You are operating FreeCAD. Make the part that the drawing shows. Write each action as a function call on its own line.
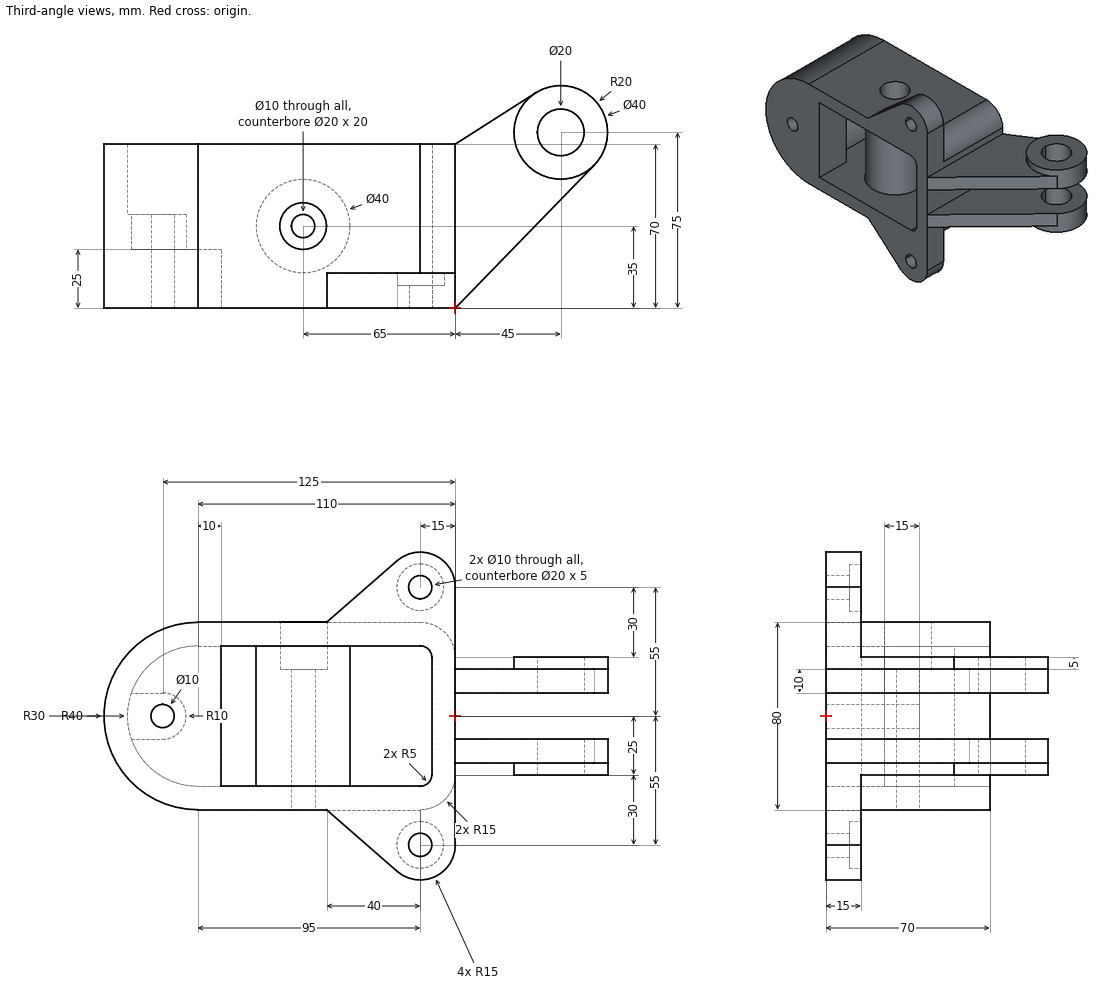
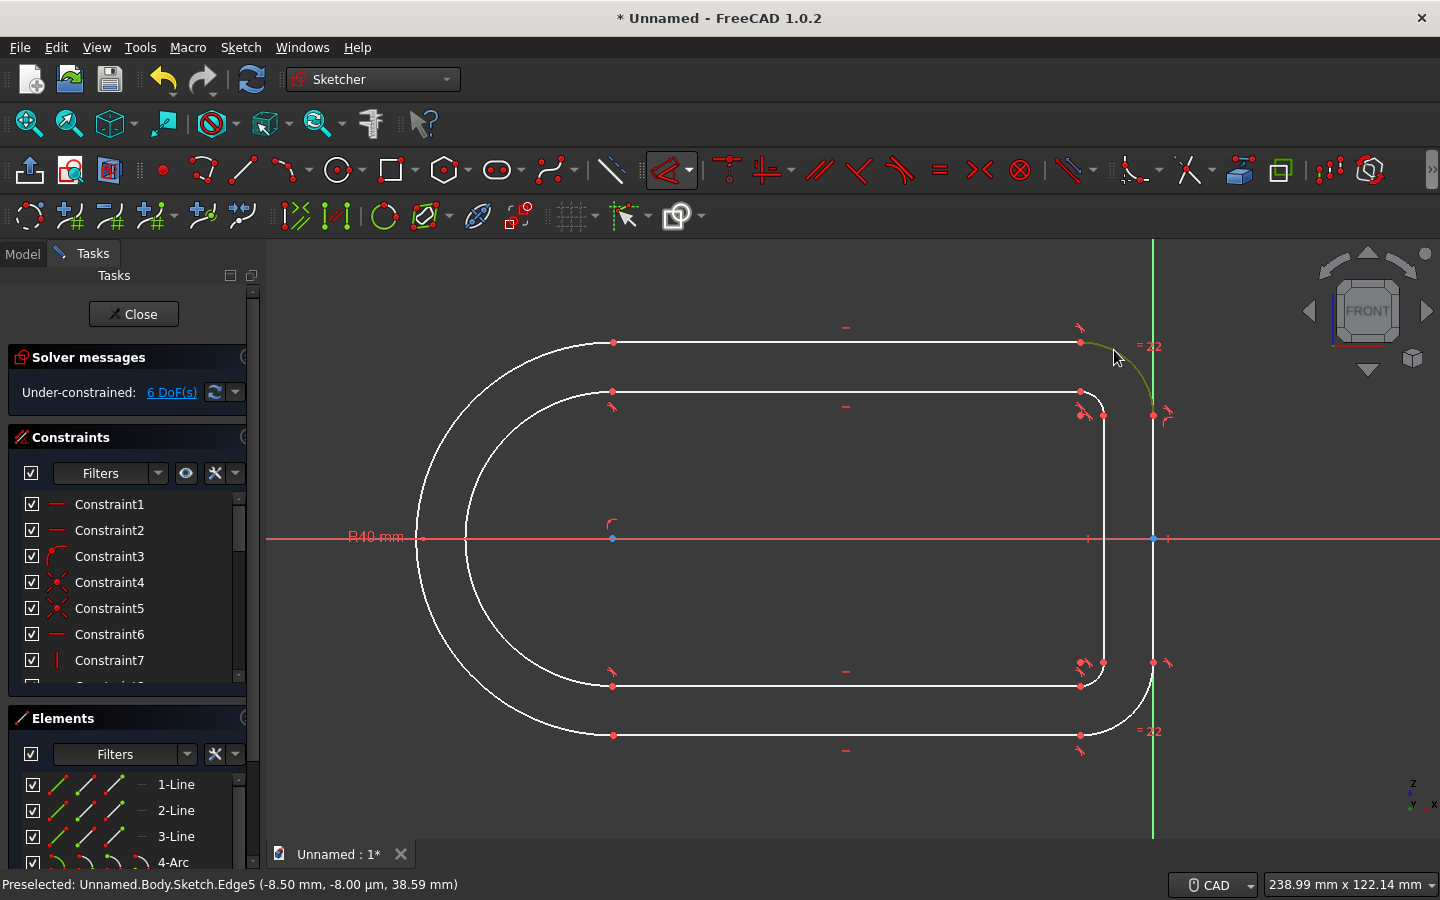
key(k)
key(r)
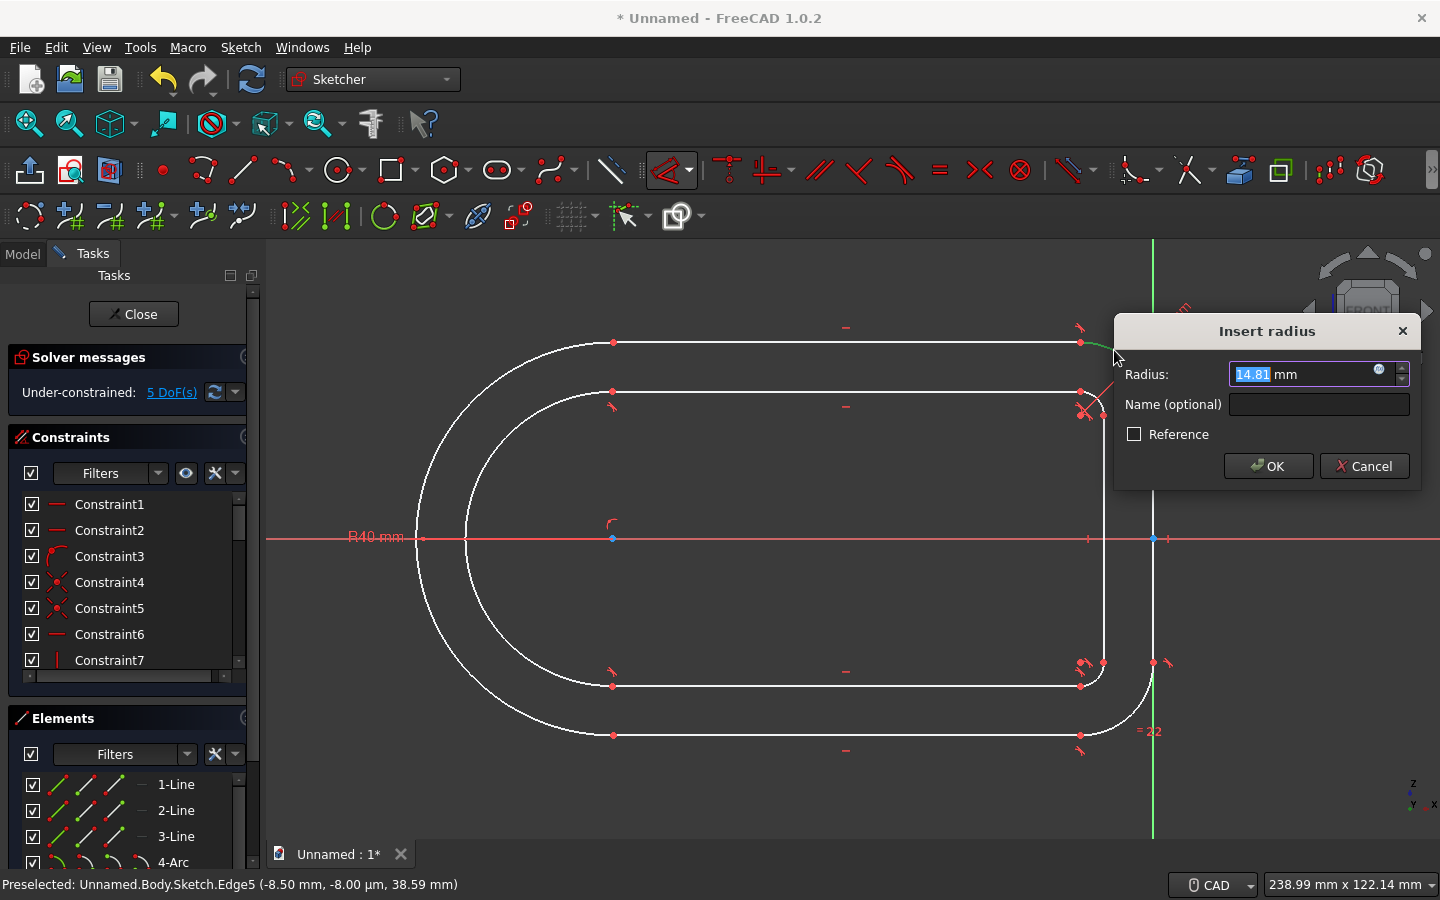
text(15)
key(Return)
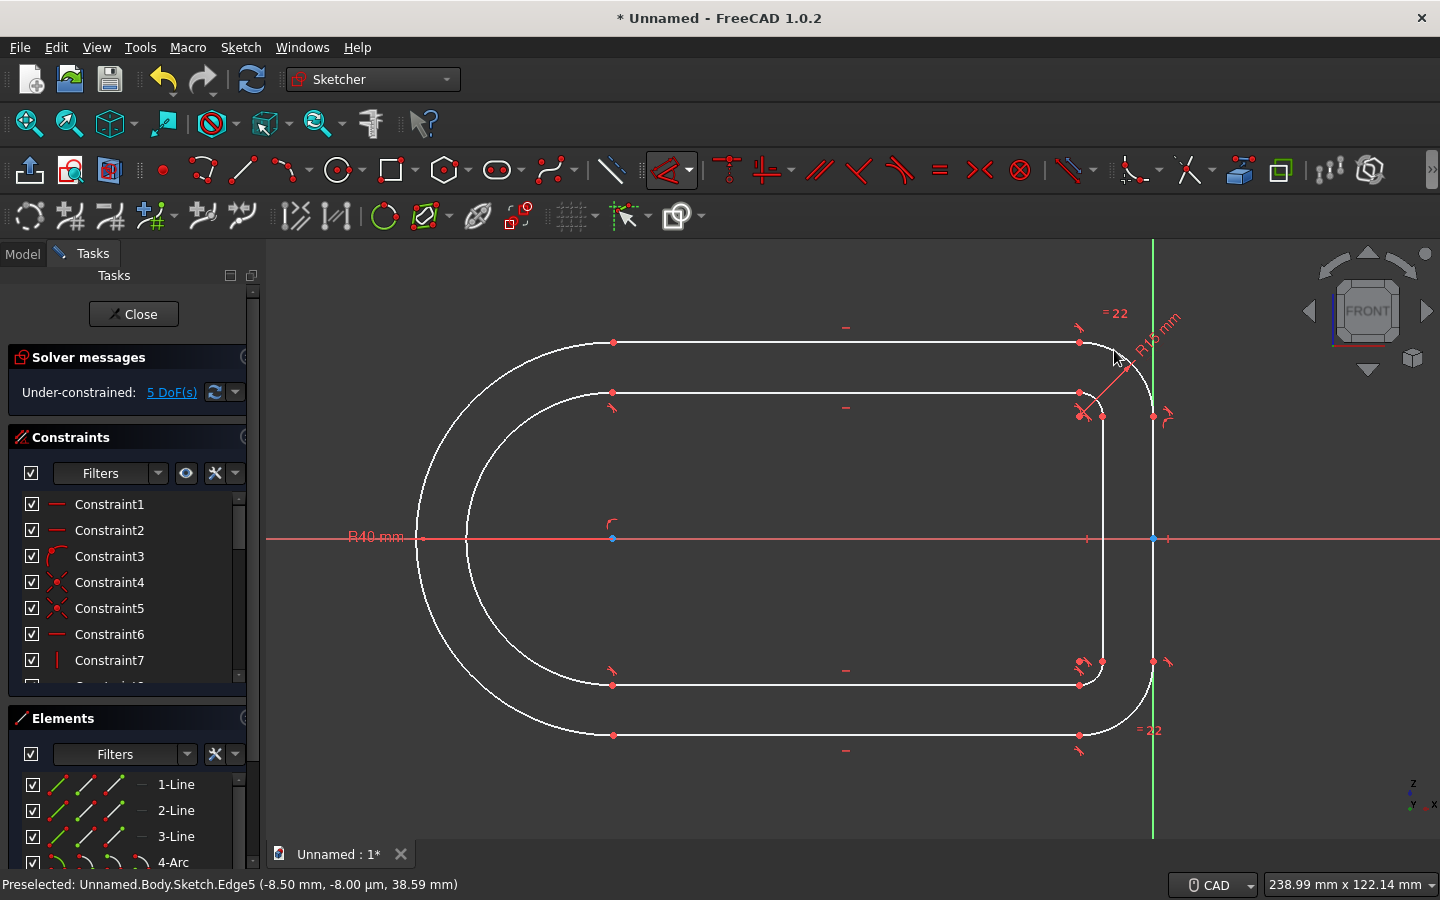
scroll(1090, 683, up, 3)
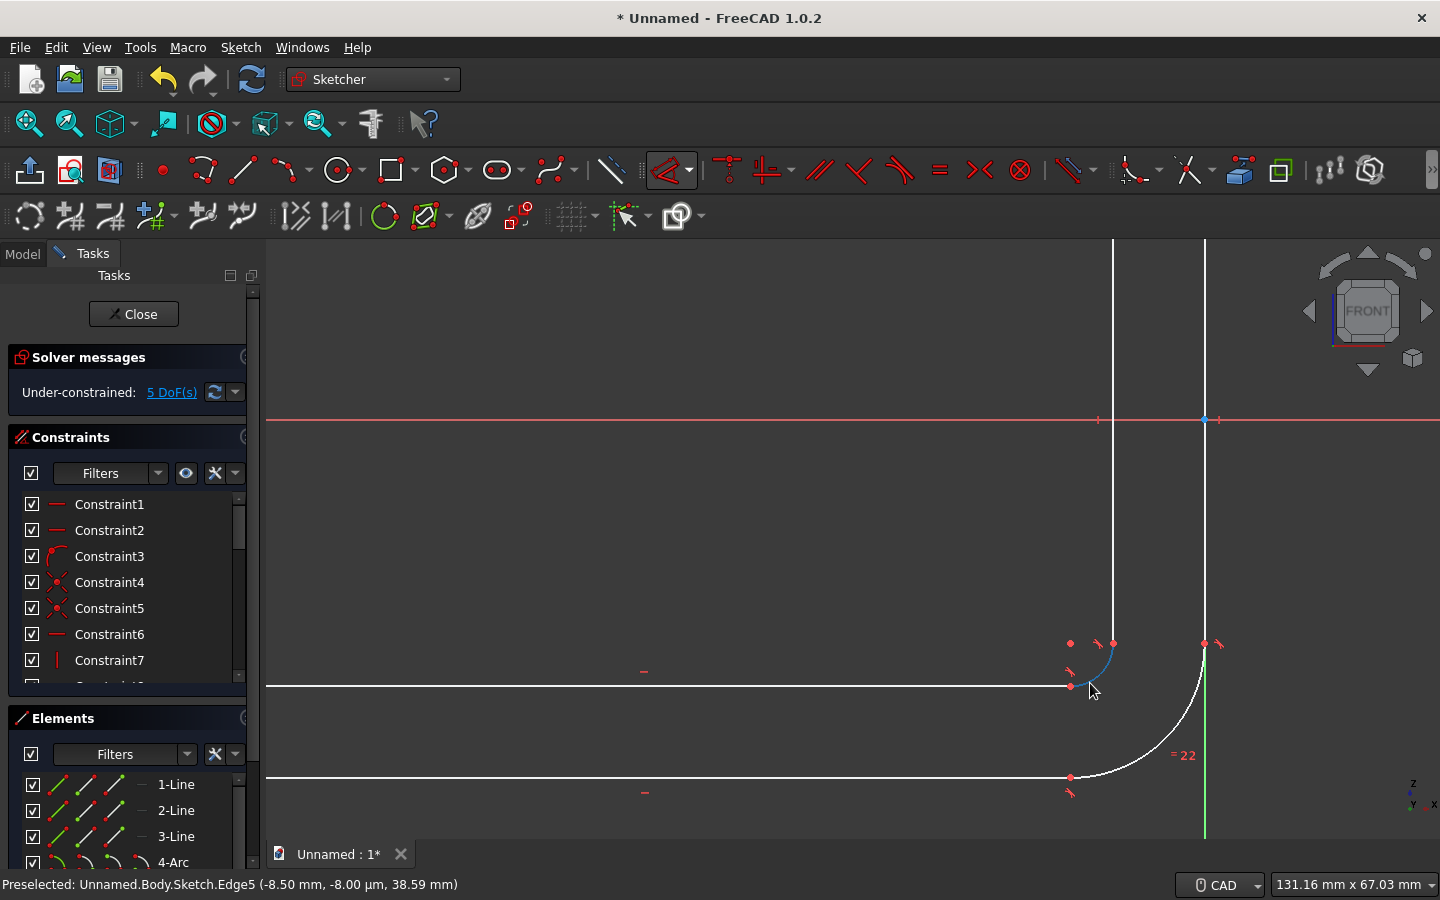
click(1090, 682)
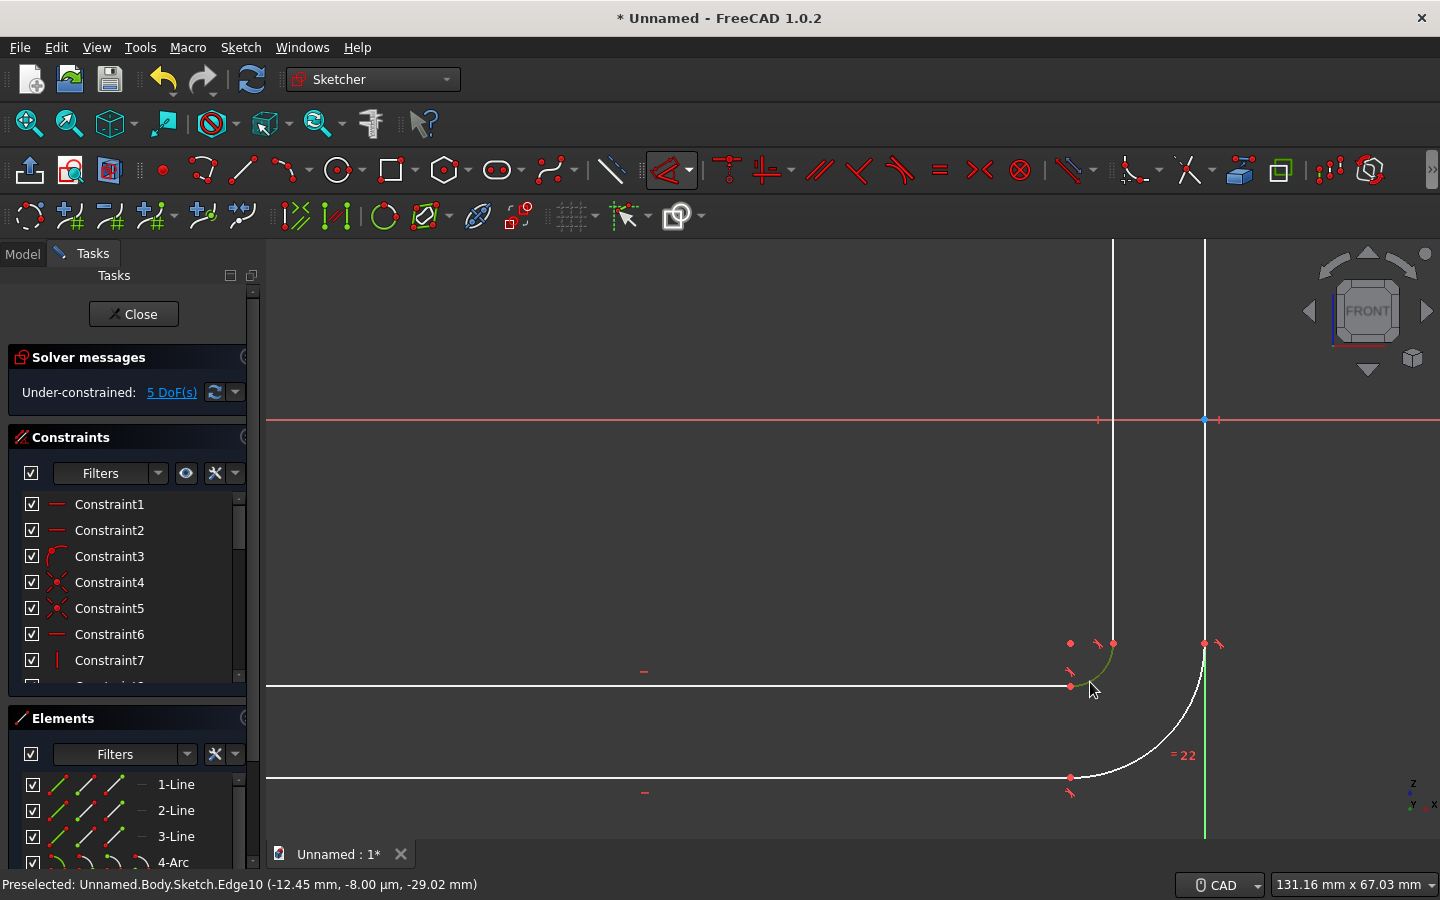
key(k)
key(r)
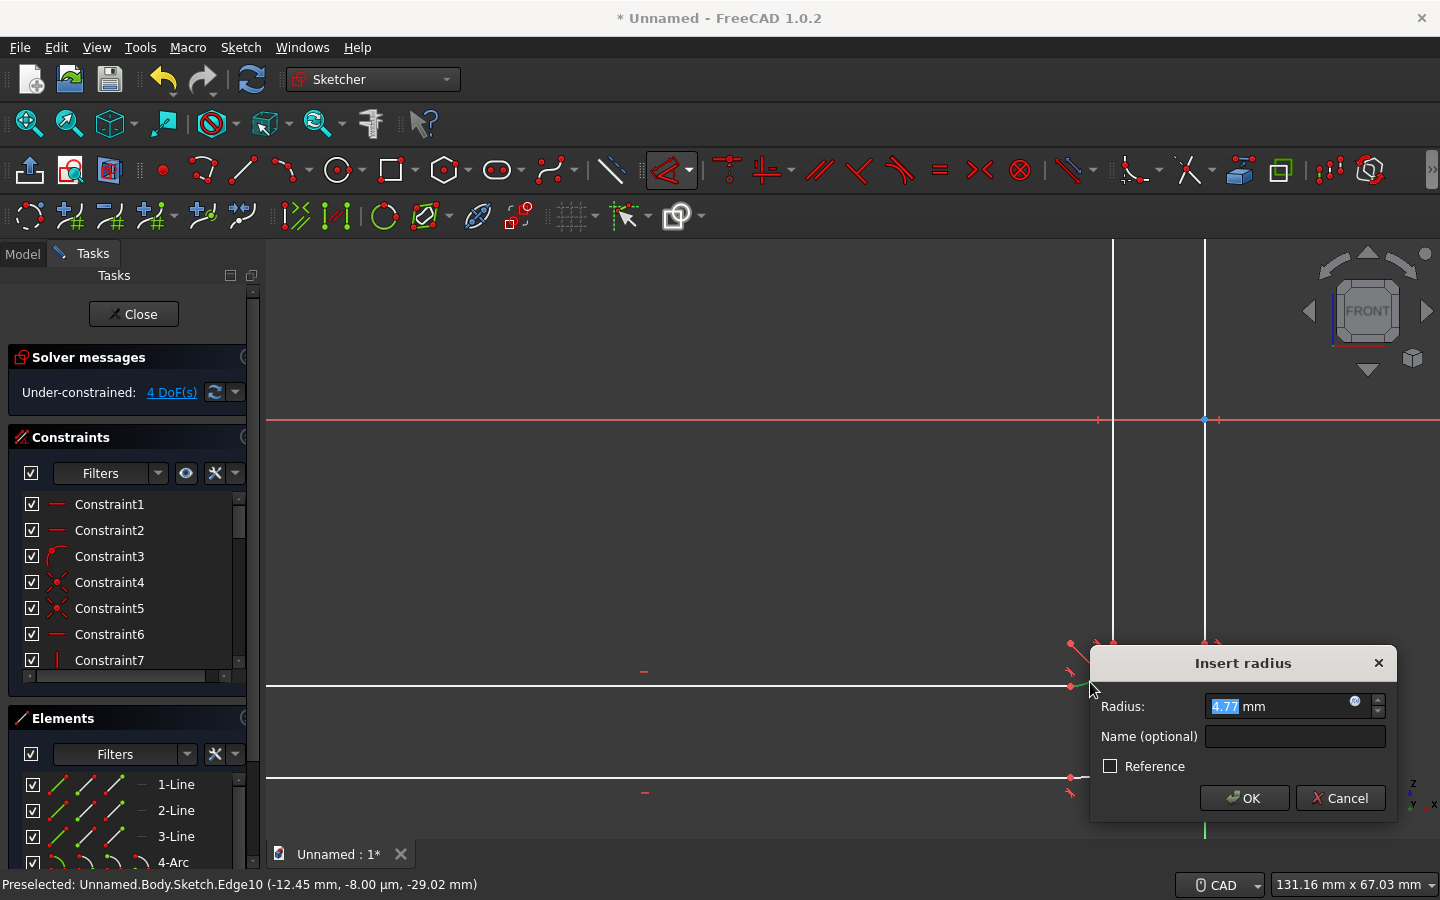
text(5)
key(Return)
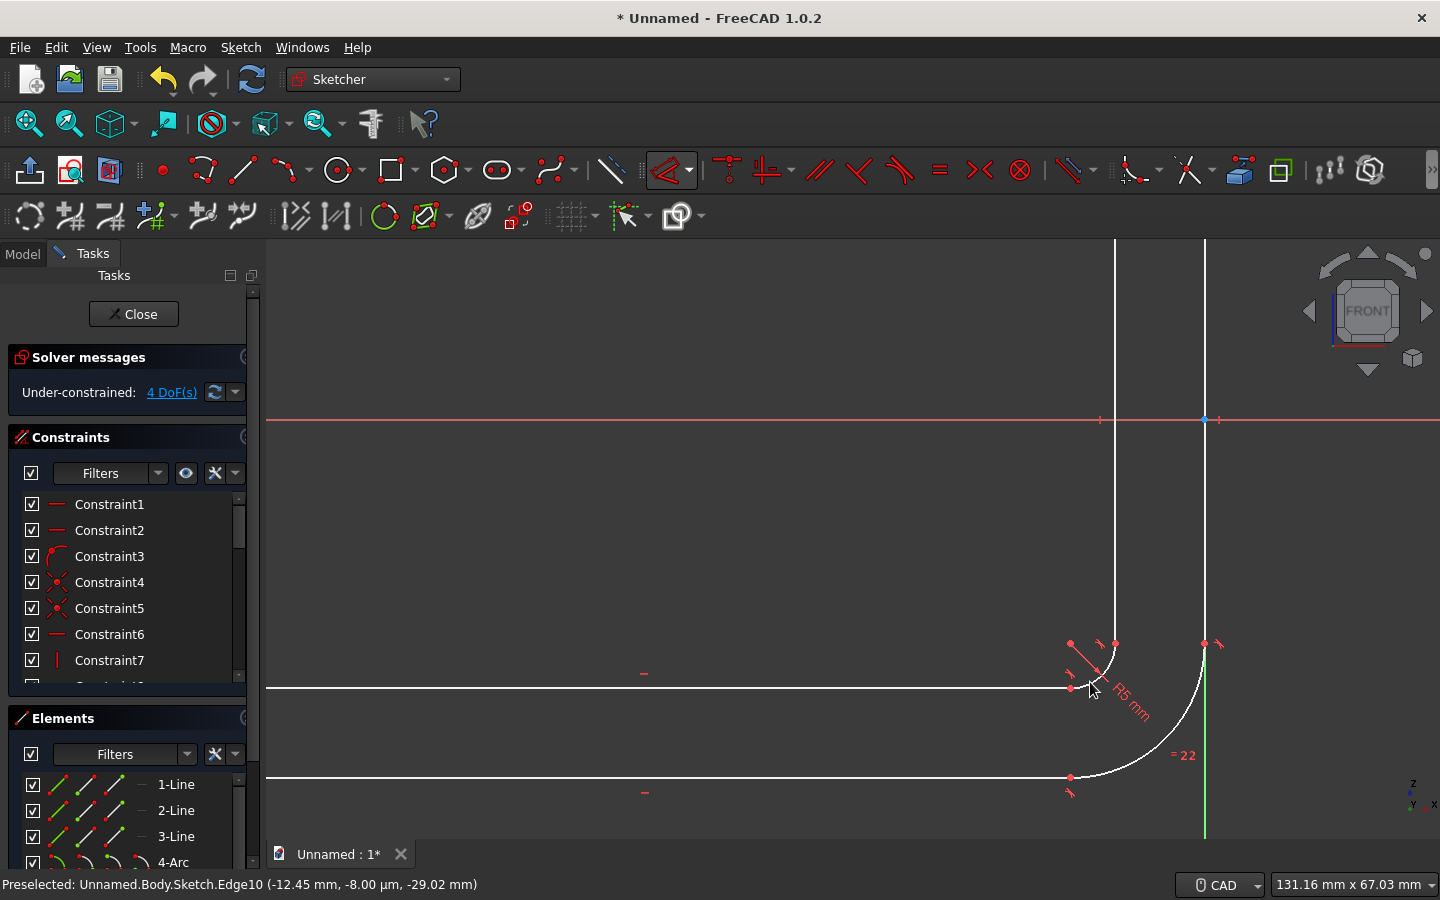
click(816, 778)